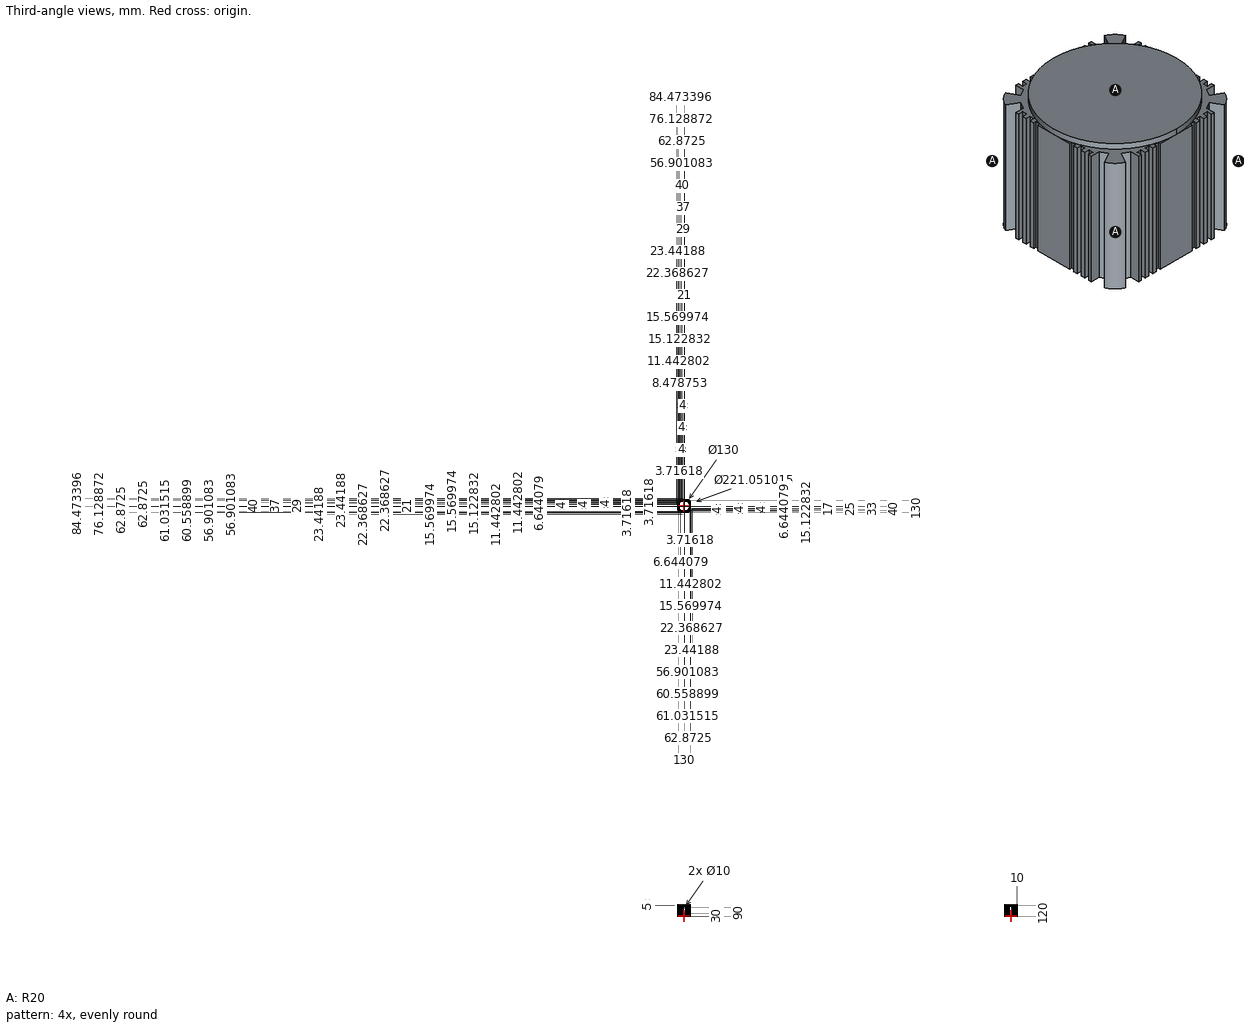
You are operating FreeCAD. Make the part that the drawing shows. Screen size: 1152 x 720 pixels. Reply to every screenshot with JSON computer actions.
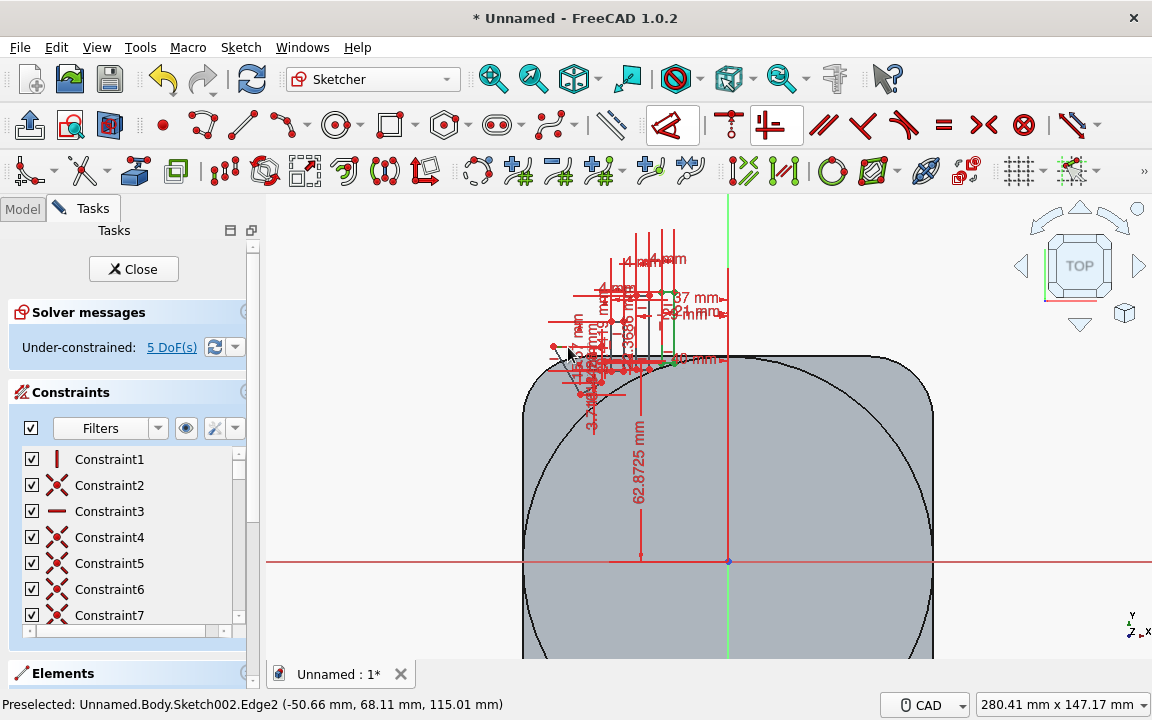
{"action": "left_click", "coordinate": [694, 126]}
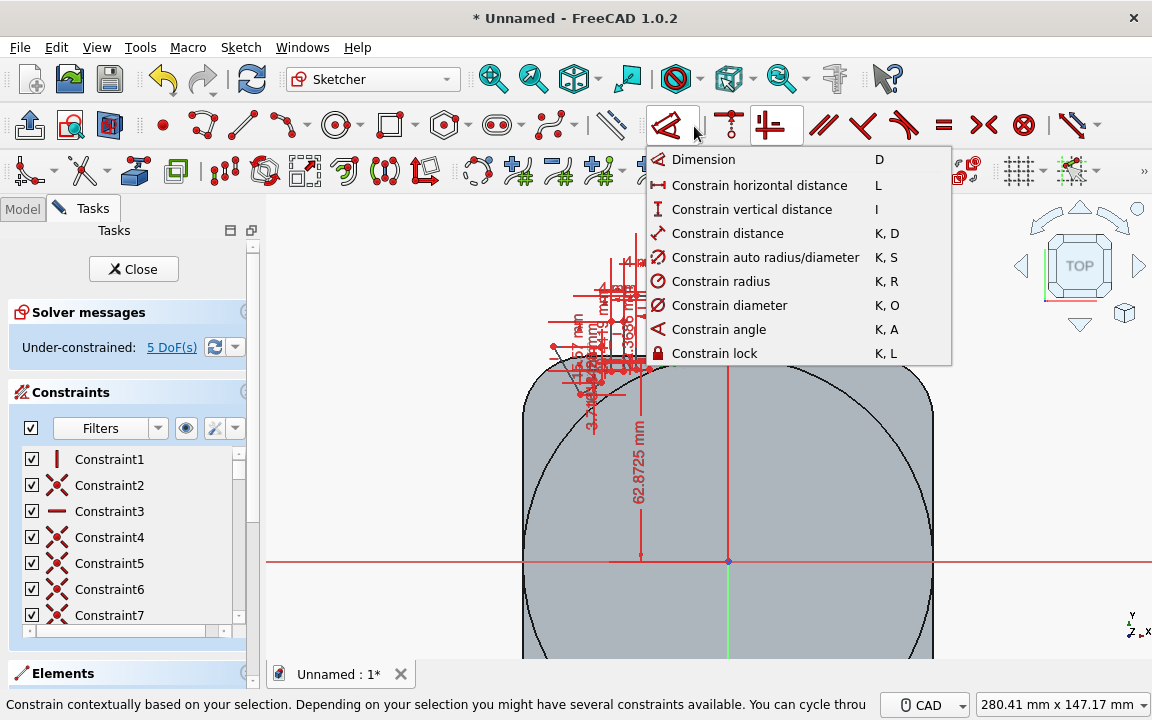
{"action": "left_click", "coordinate": [799, 185]}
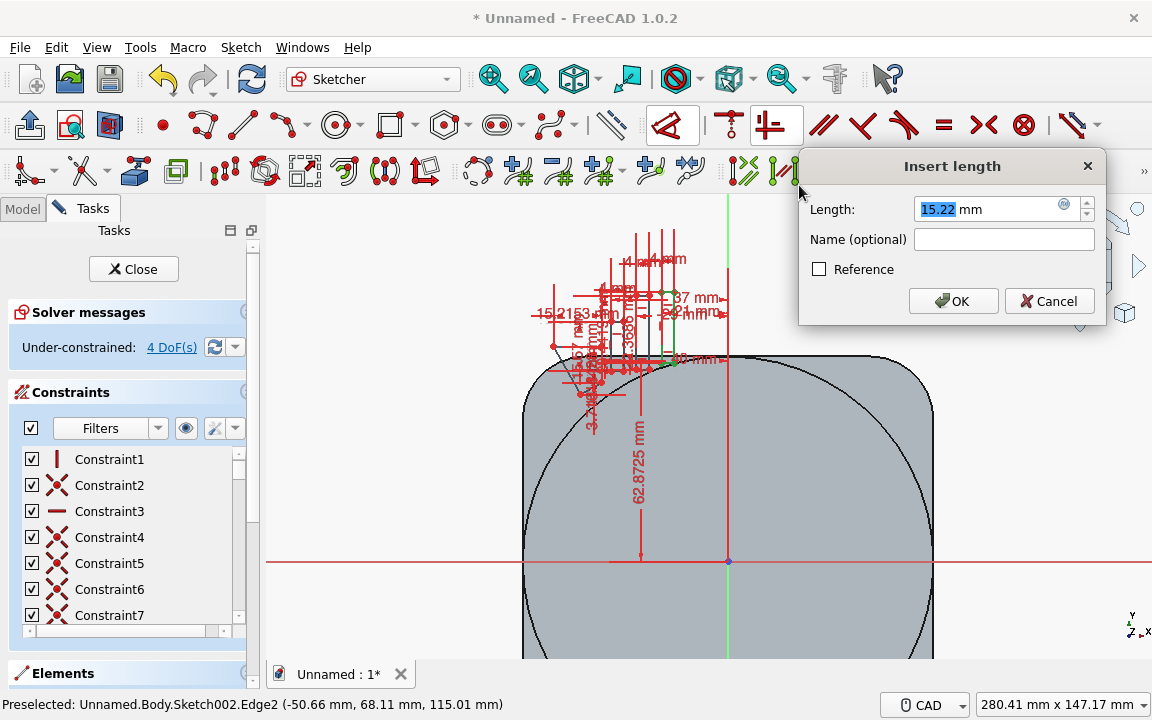
{"action": "type", "text": "15.122832"}
{"action": "key", "text": "Return"}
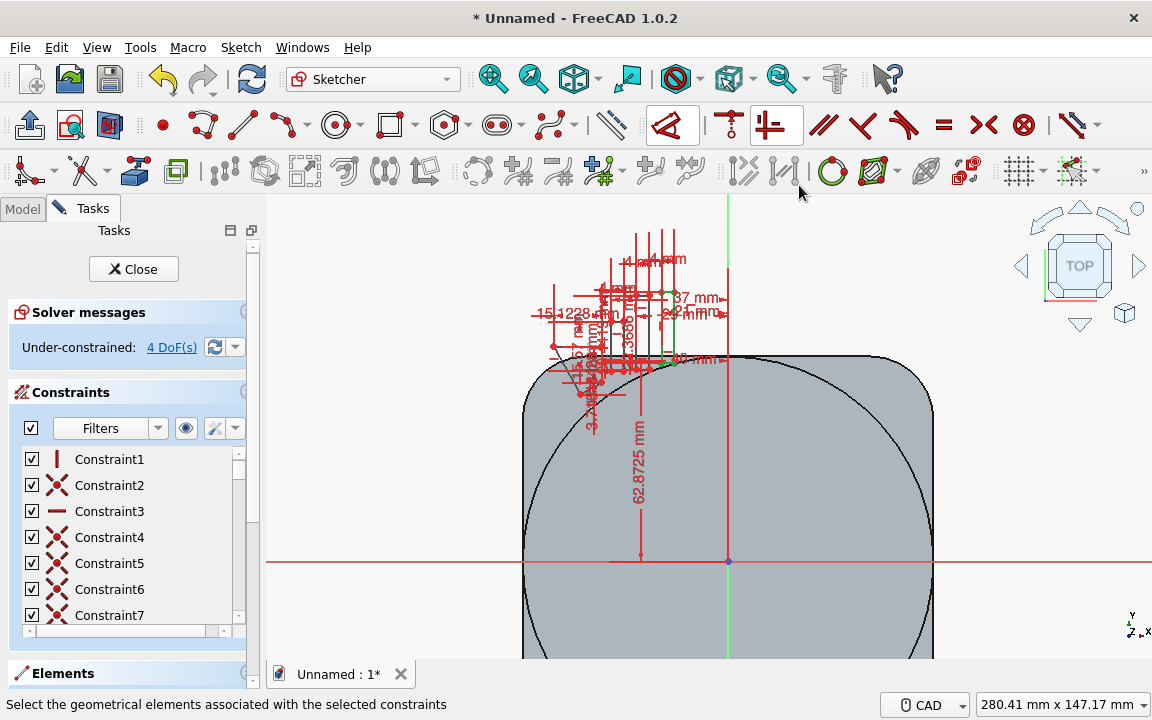
{"action": "scroll", "coordinate": [562, 361], "scroll_direction": "up", "scroll_amount": 2}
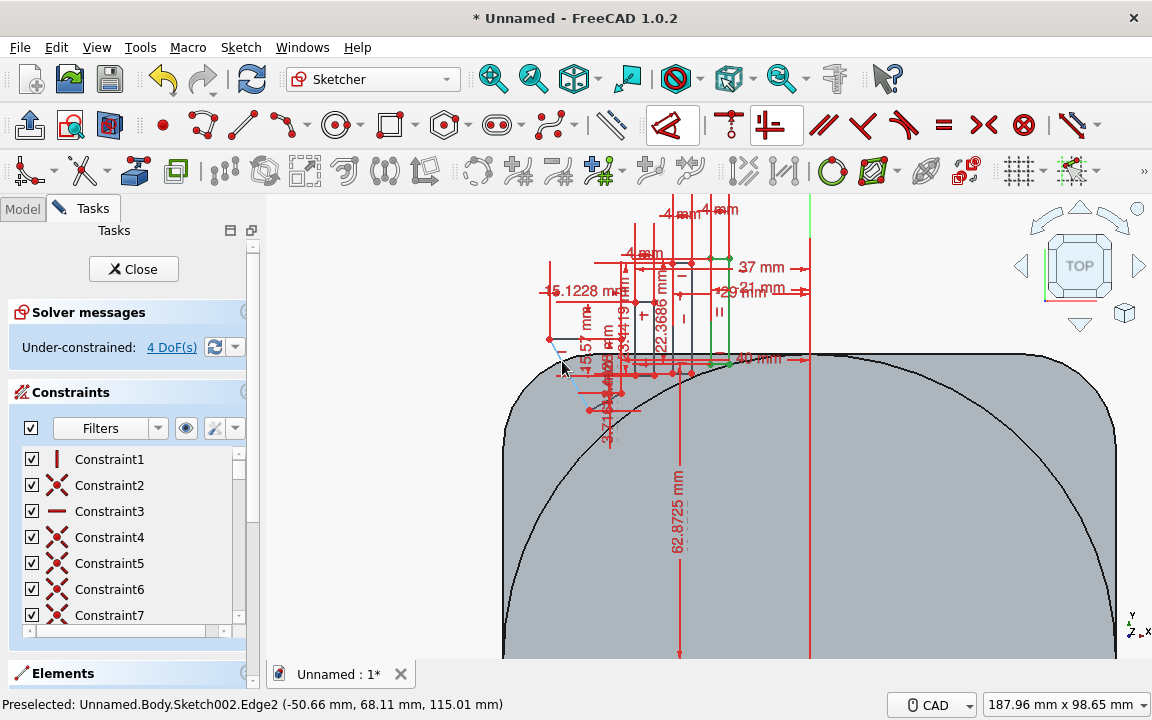
{"action": "left_click", "coordinate": [562, 361]}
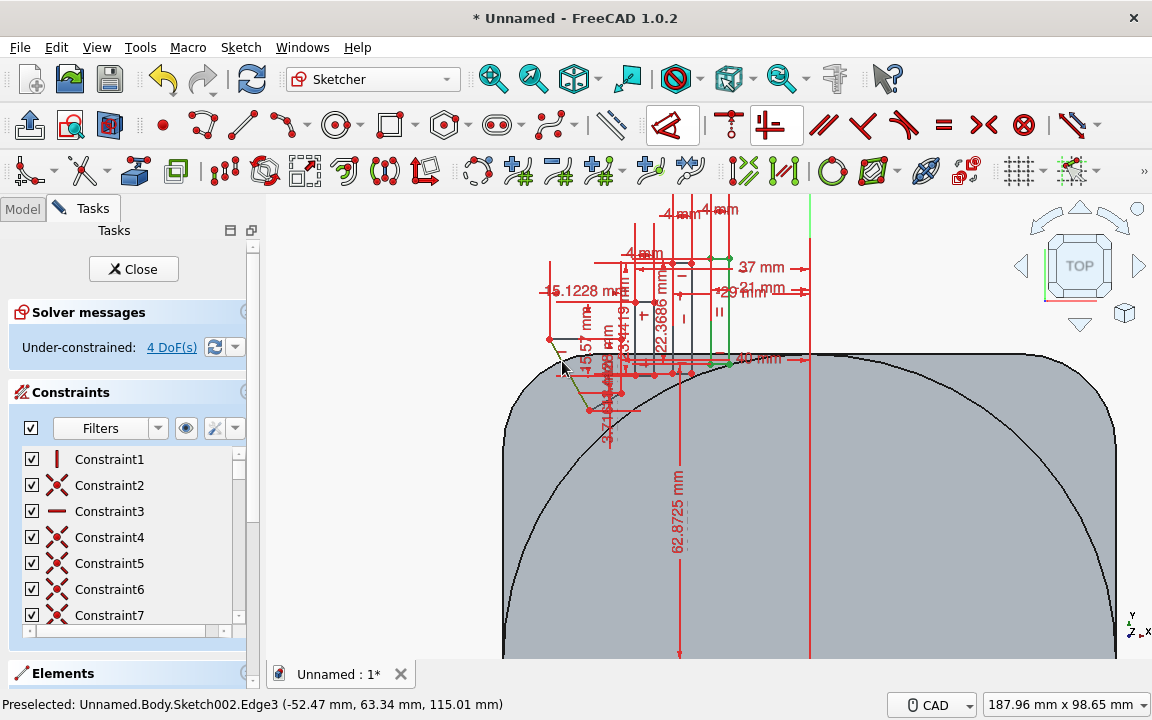
{"action": "key", "text": "l"}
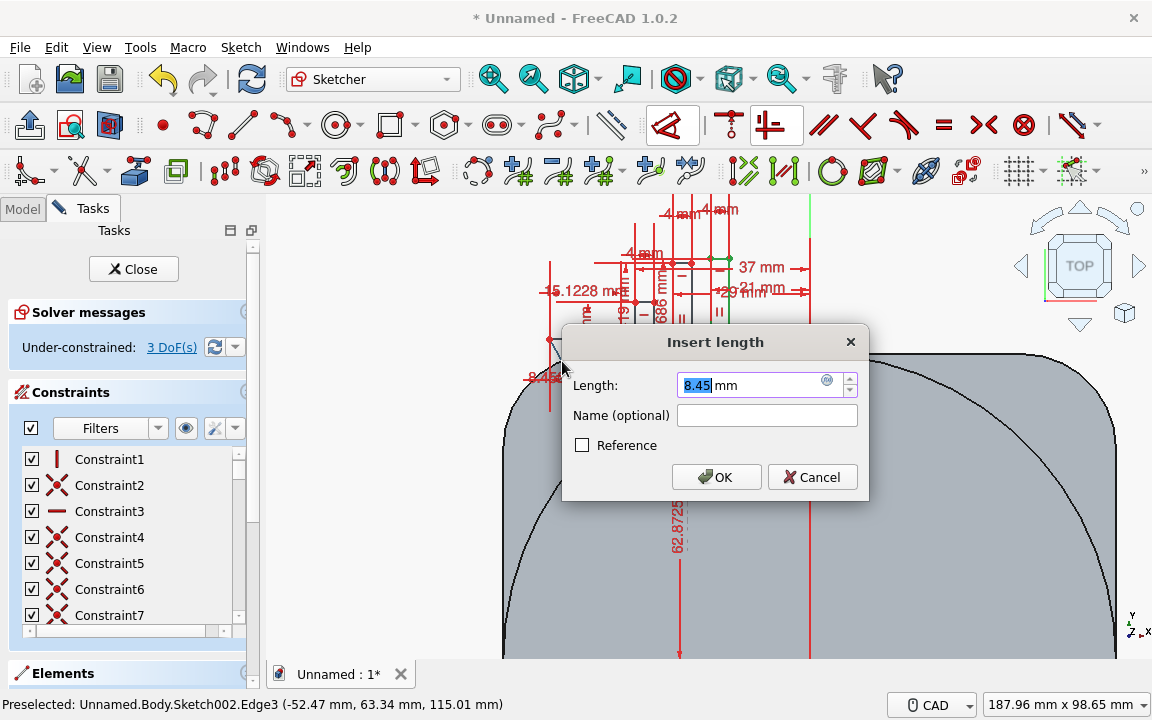
{"action": "type", "text": "8.478753"}
{"action": "key", "text": "Return"}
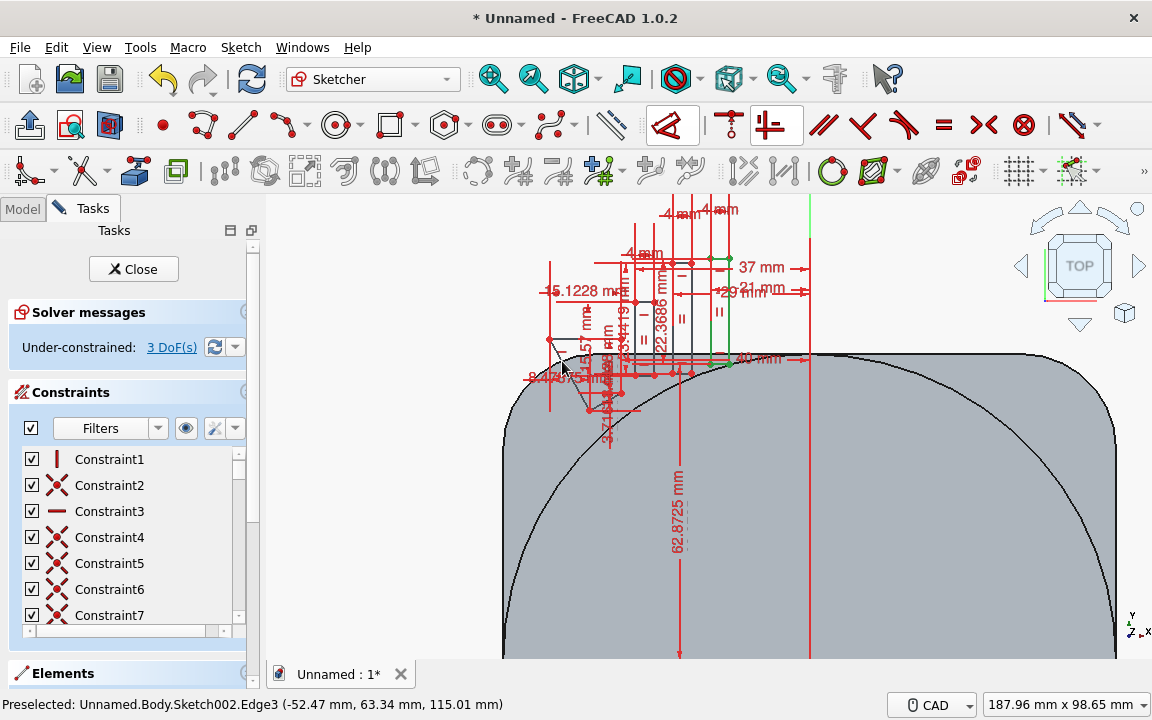
{"action": "left_click", "coordinate": [621, 393]}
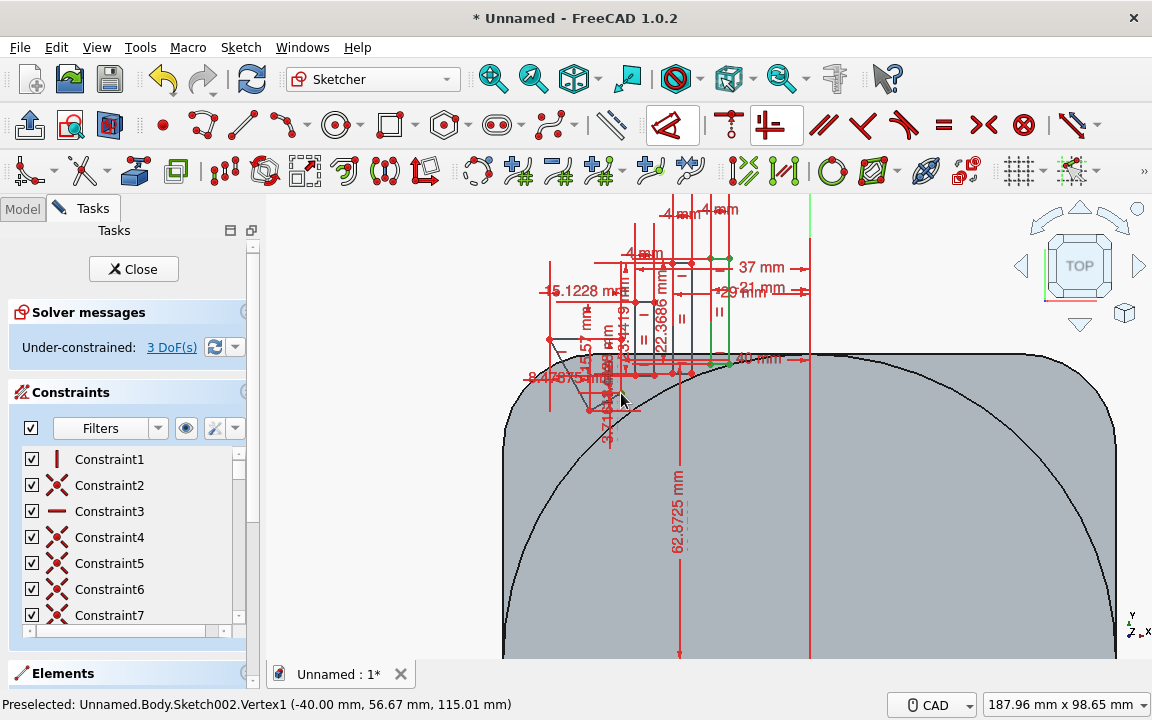
{"action": "left_click", "coordinate": [694, 126]}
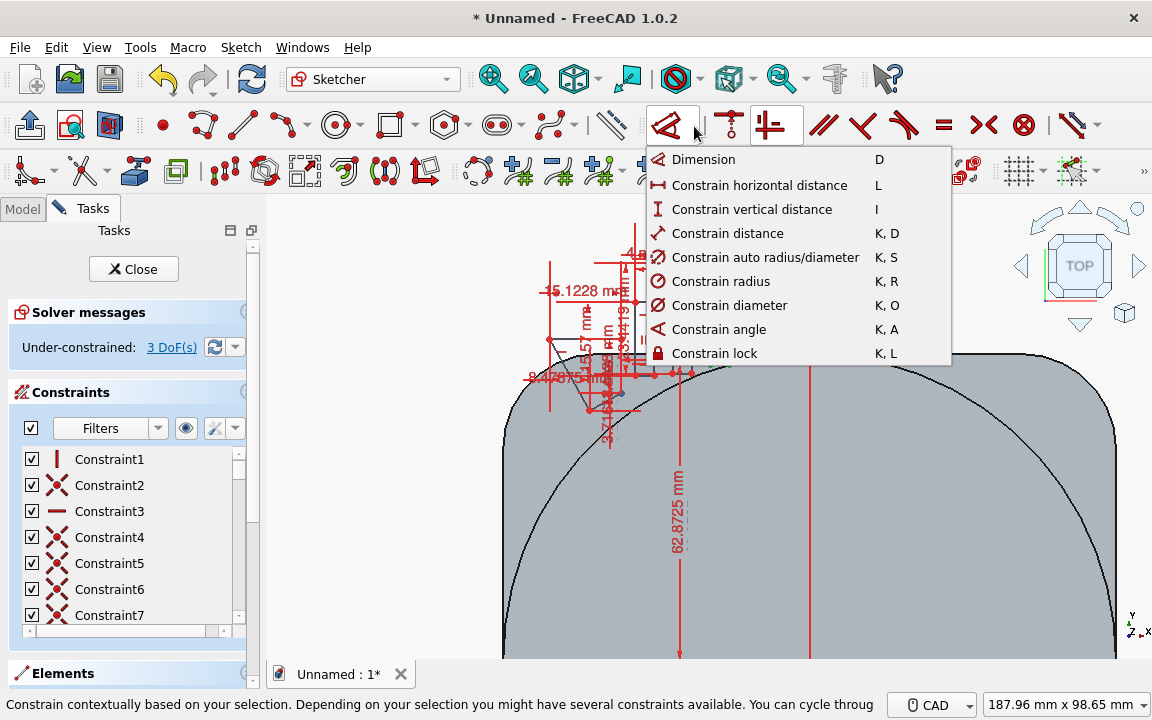
{"action": "left_click", "coordinate": [799, 209]}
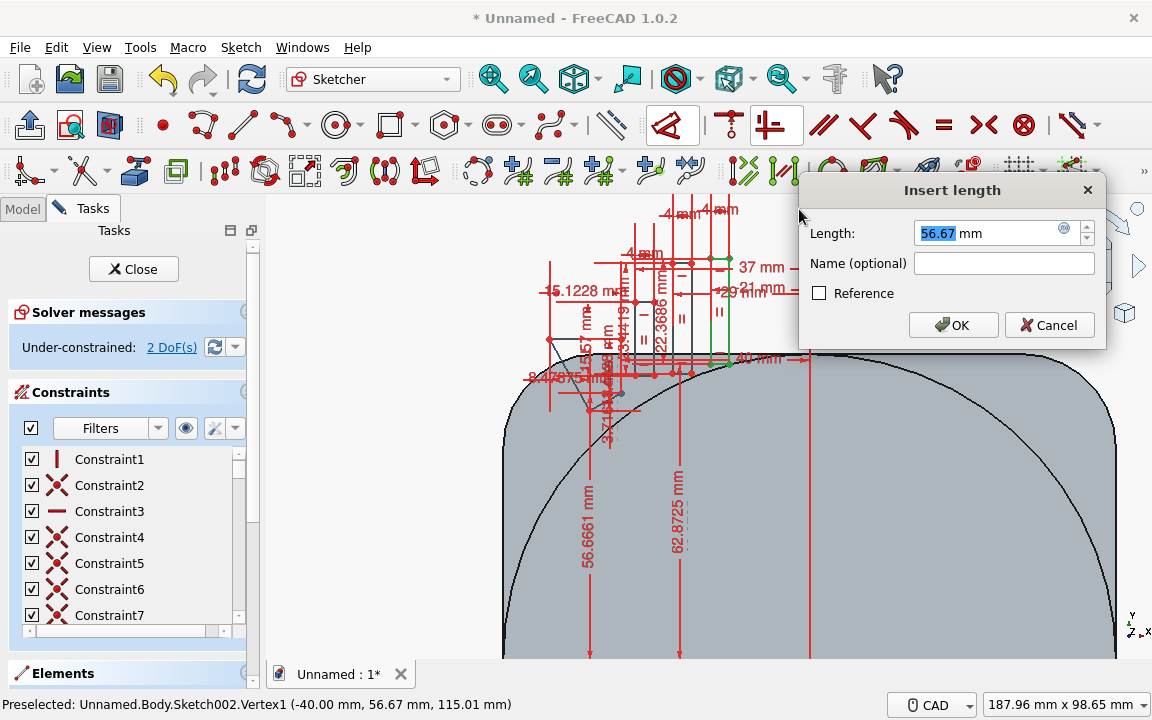
{"action": "type", "text": "56.901083"}
{"action": "key", "text": "Return"}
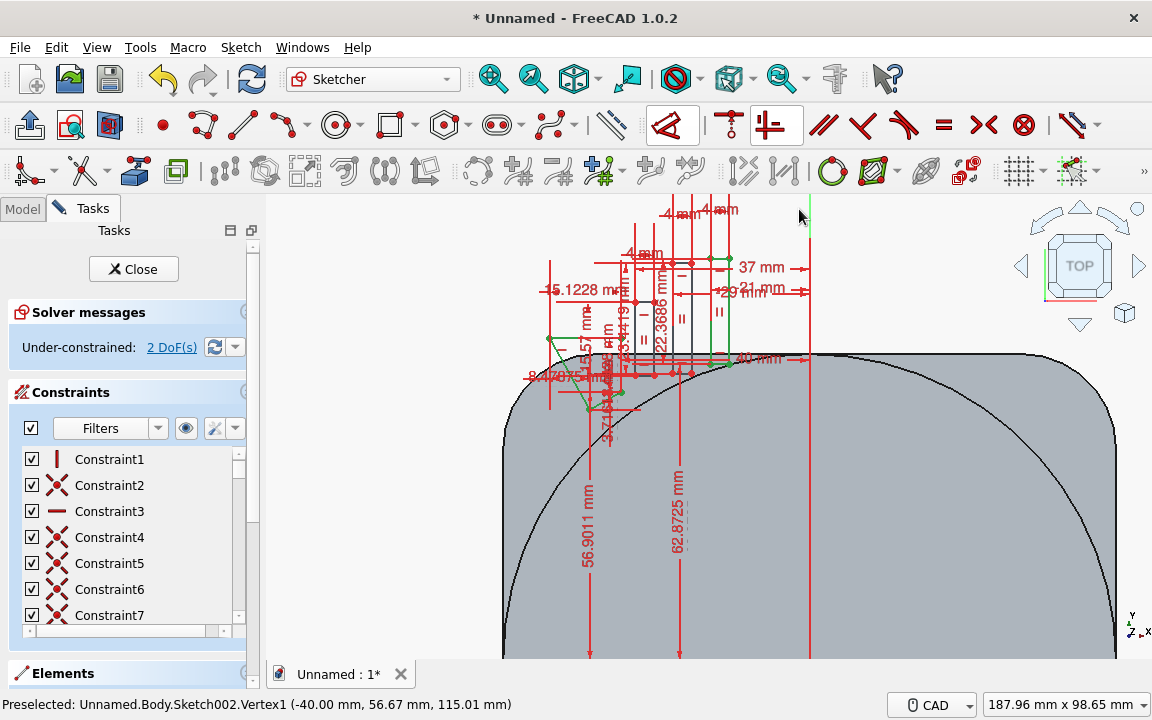
{"action": "left_click", "coordinate": [635, 302]}